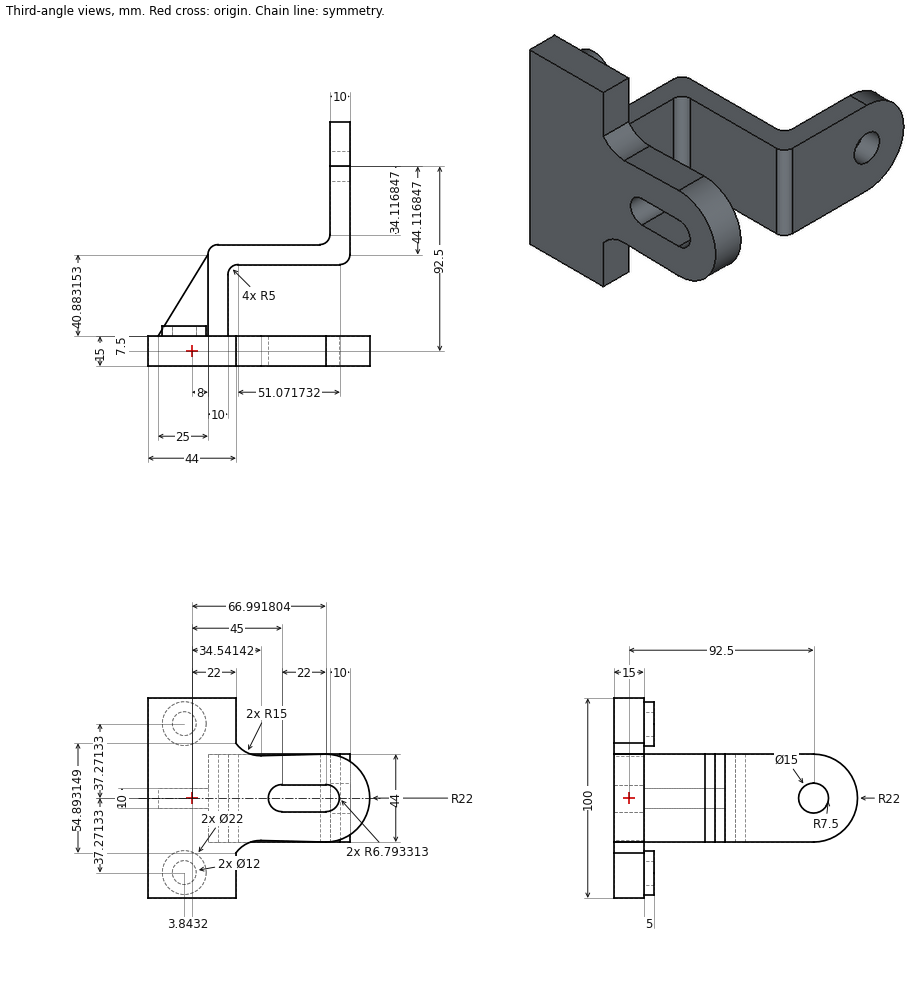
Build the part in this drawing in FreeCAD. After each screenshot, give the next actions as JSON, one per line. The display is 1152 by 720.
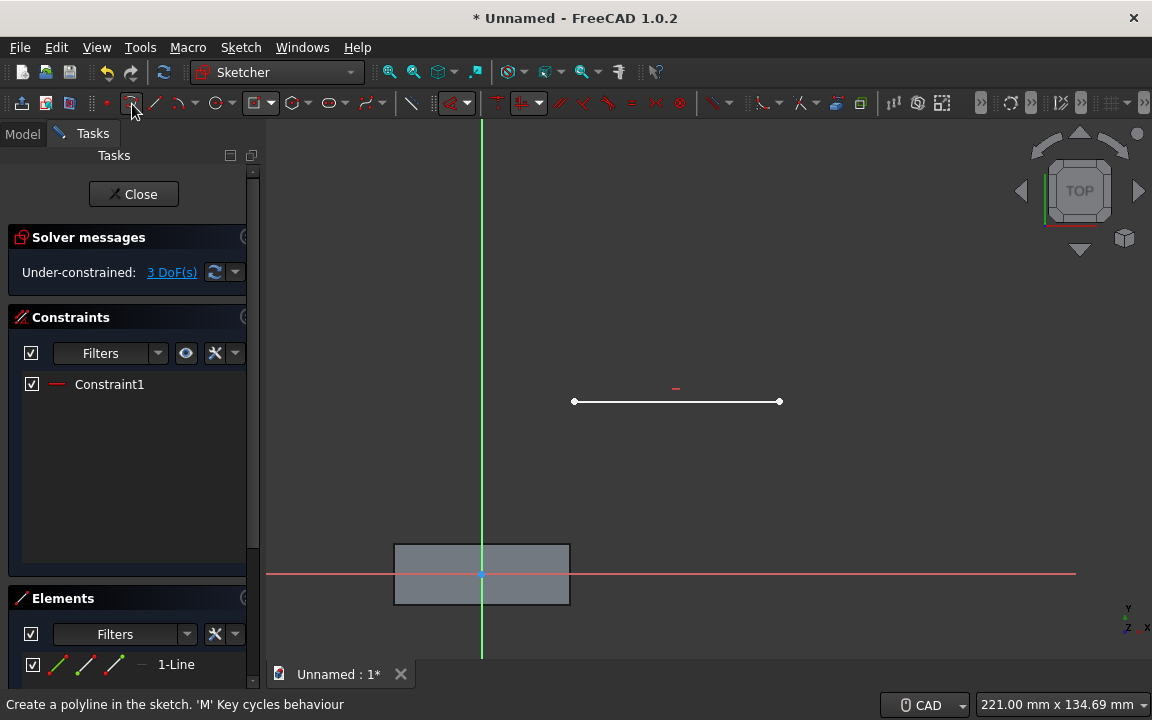
{"action": "left_click", "coordinate": [799, 380]}
{"action": "left_click", "coordinate": [799, 204]}
{"action": "left_click", "coordinate": [759, 204]}
{"action": "left_click", "coordinate": [759, 340]}
{"action": "right_click", "coordinate": [759, 340]}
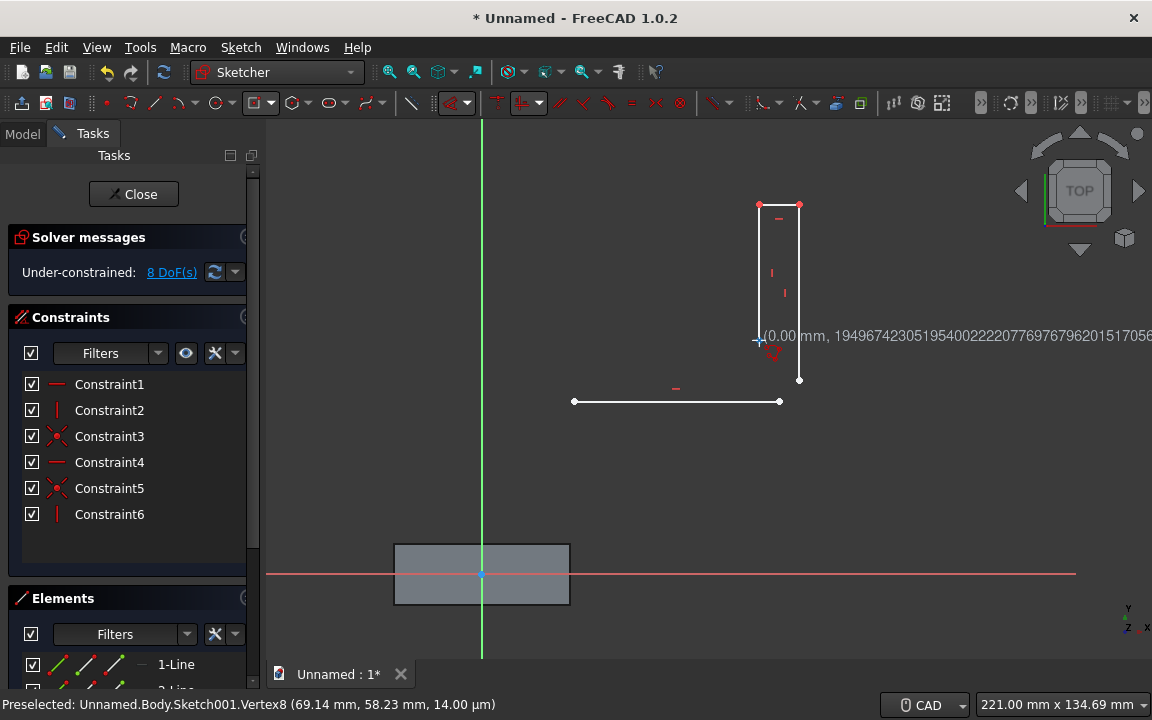
{"action": "left_click", "coordinate": [156, 104]}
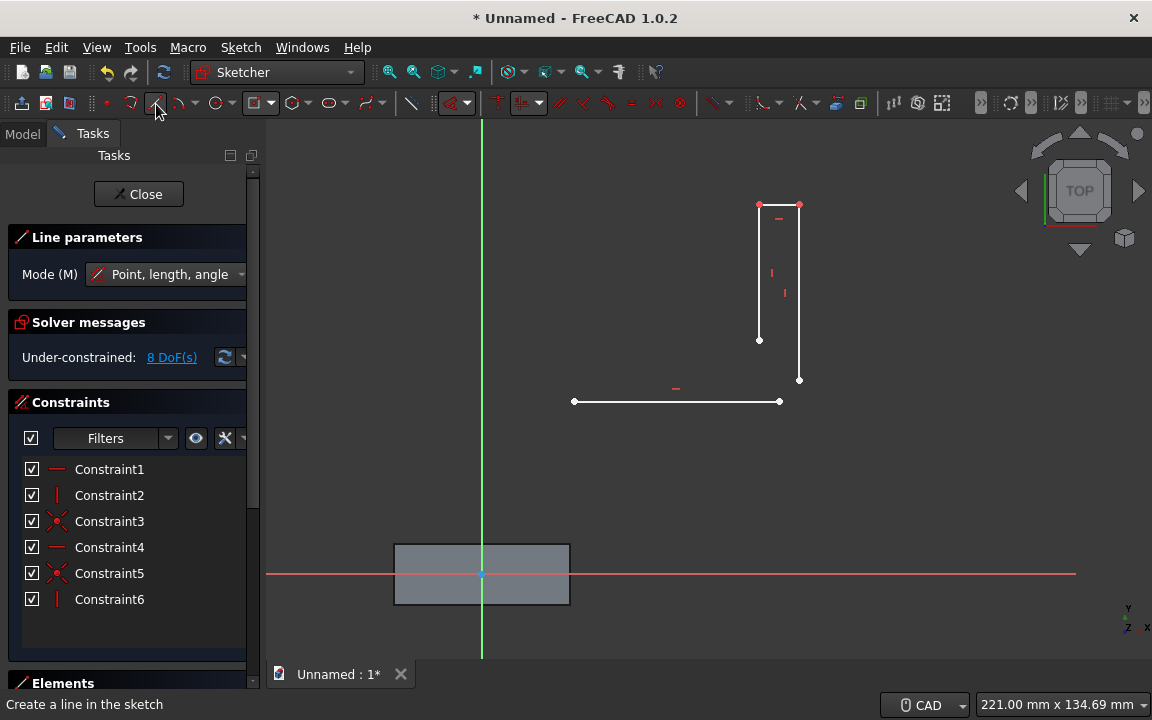
{"action": "left_click", "coordinate": [739, 360]}
{"action": "left_click", "coordinate": [534, 360]}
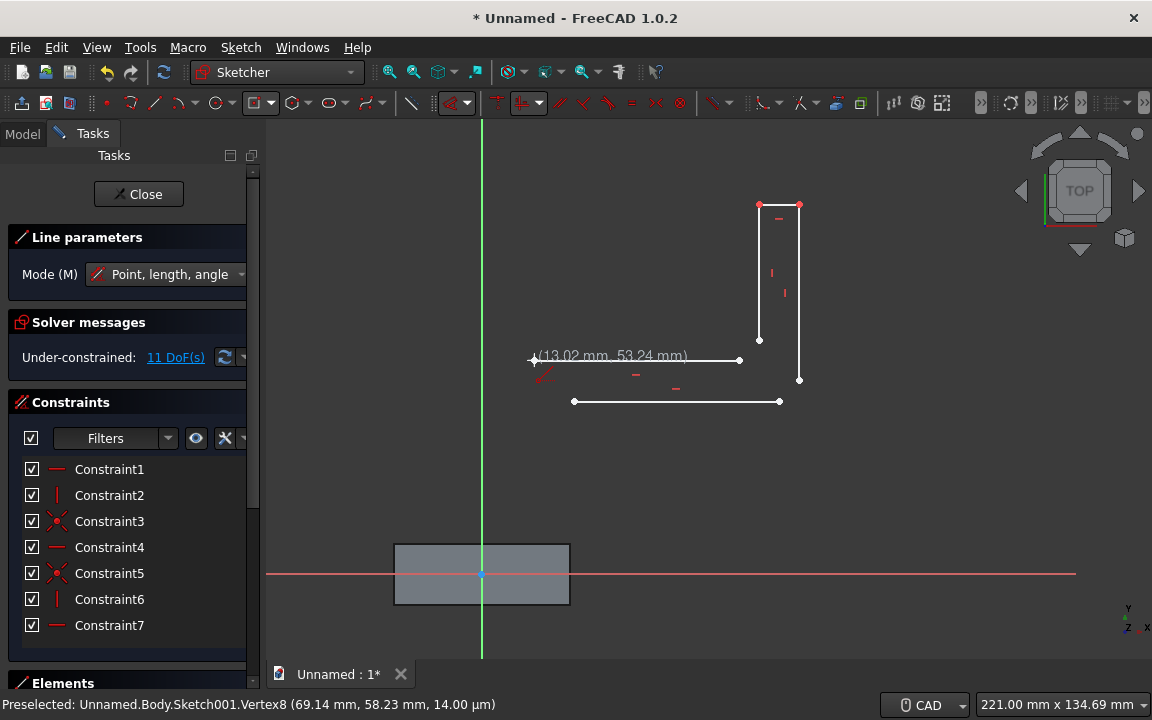
{"action": "left_click", "coordinate": [132, 104]}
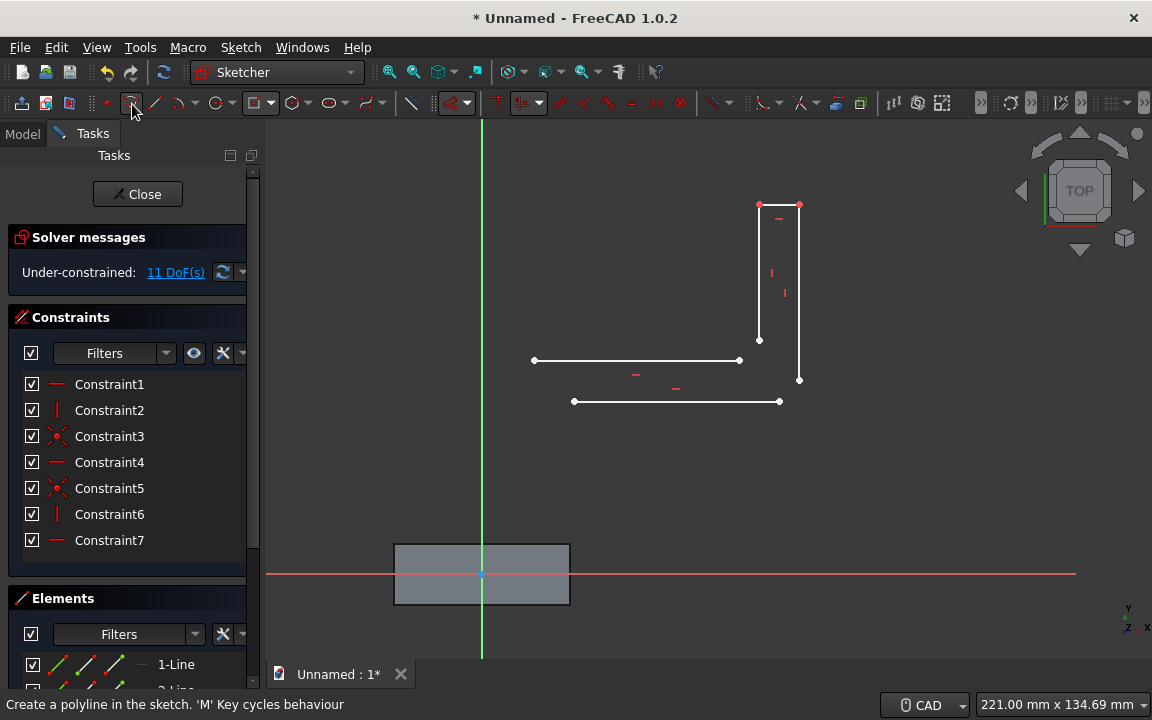
{"action": "left_click", "coordinate": [514, 380]}
{"action": "left_click", "coordinate": [514, 544]}
{"action": "left_click", "coordinate": [554, 544]}
{"action": "left_click", "coordinate": [554, 421]}
{"action": "right_click", "coordinate": [554, 421]}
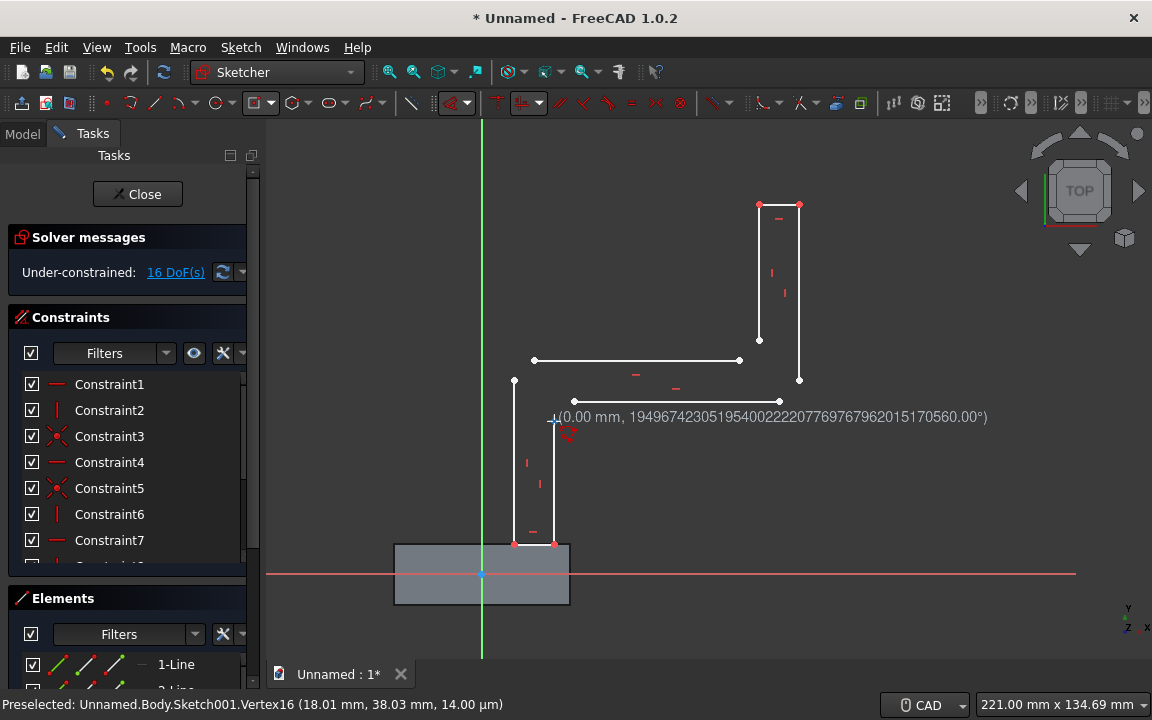
{"action": "left_click", "coordinate": [198, 104]}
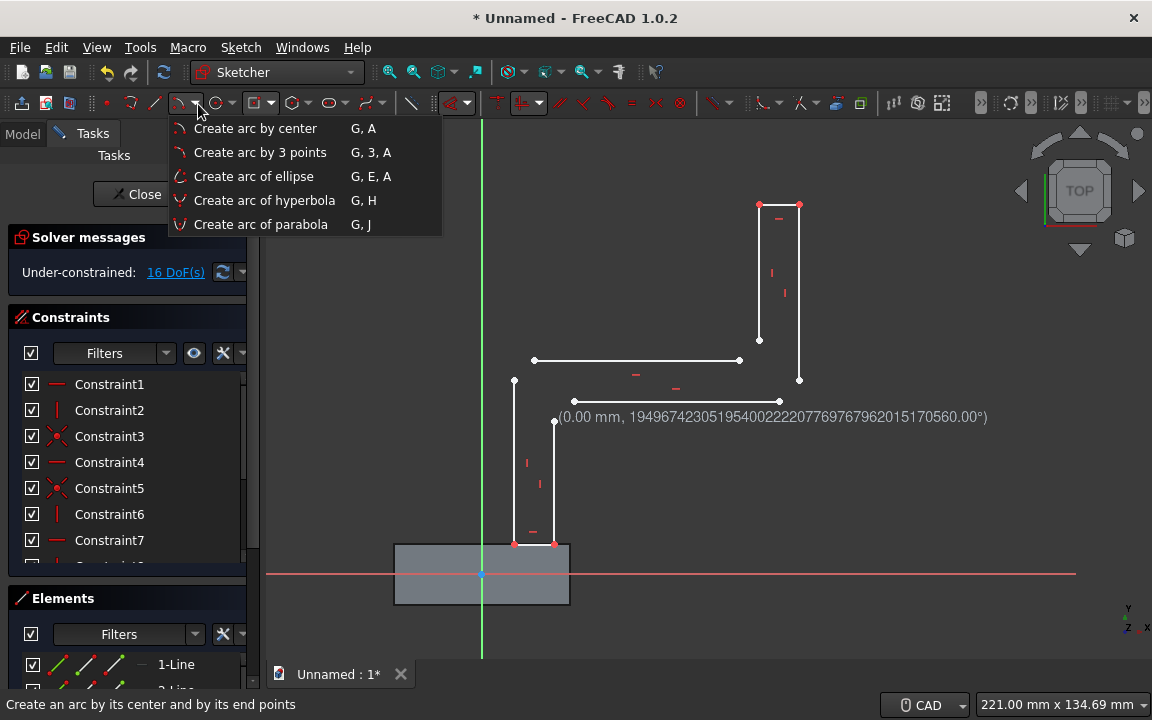
{"action": "left_click", "coordinate": [306, 152]}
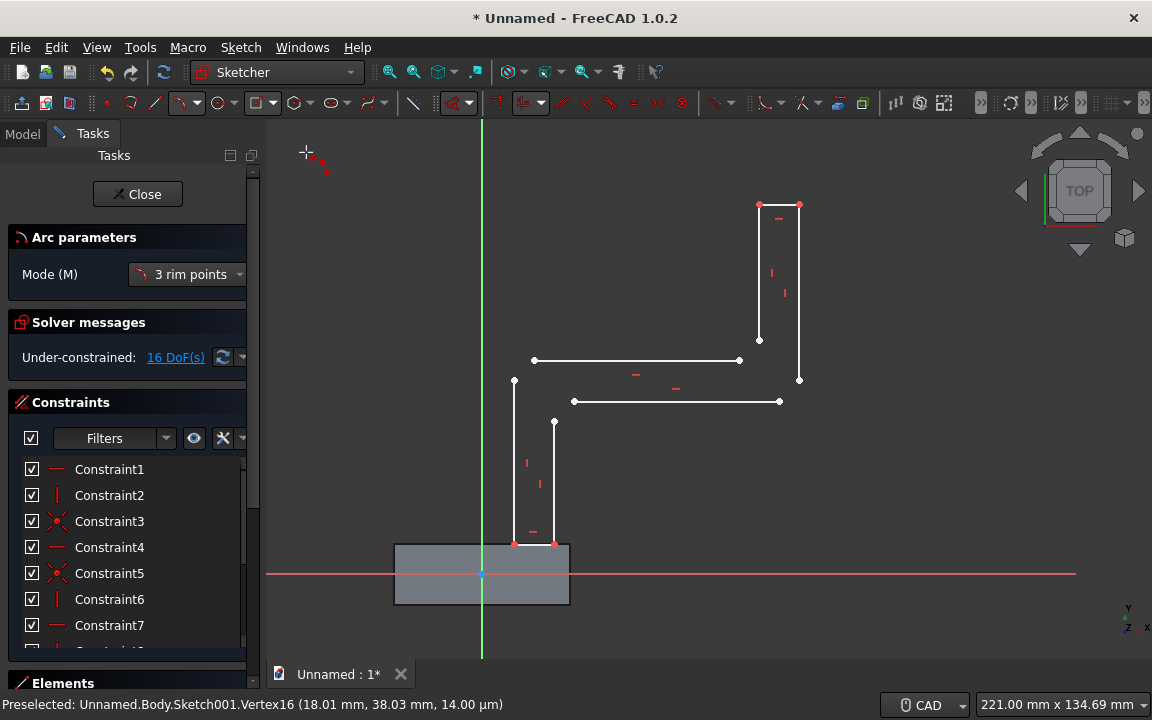
{"action": "left_click", "coordinate": [779, 402]}
{"action": "left_click", "coordinate": [799, 381]}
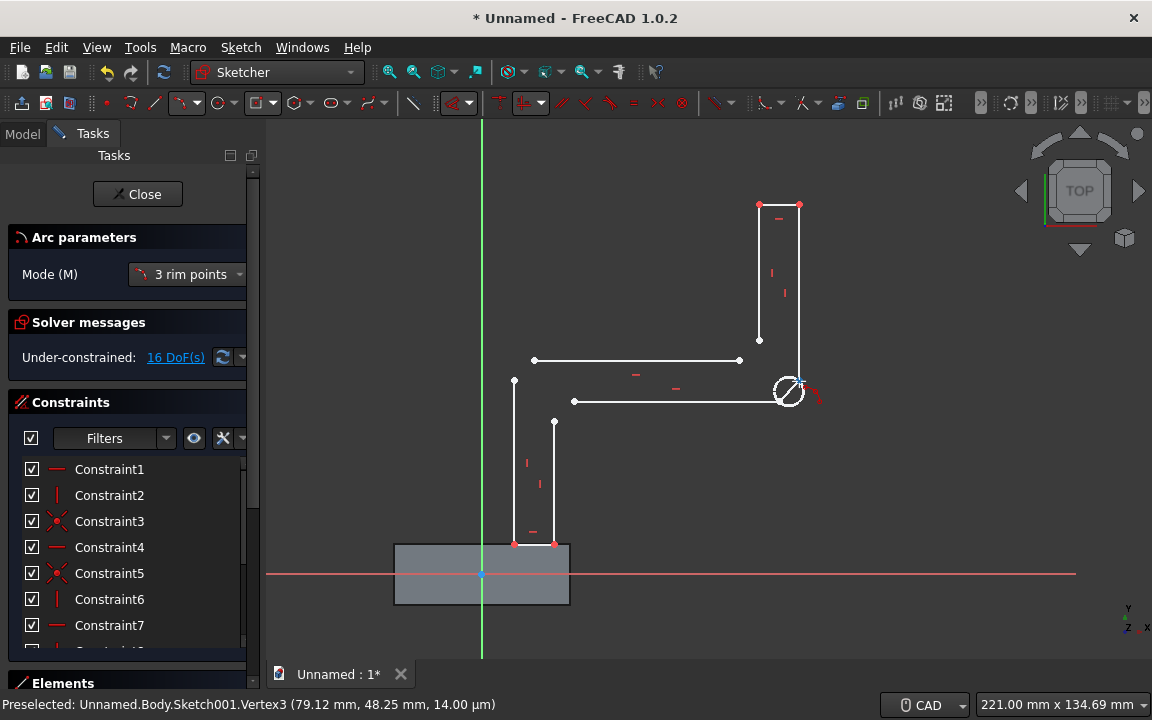
{"action": "scroll", "coordinate": [793, 395], "scroll_direction": "up", "scroll_amount": 5}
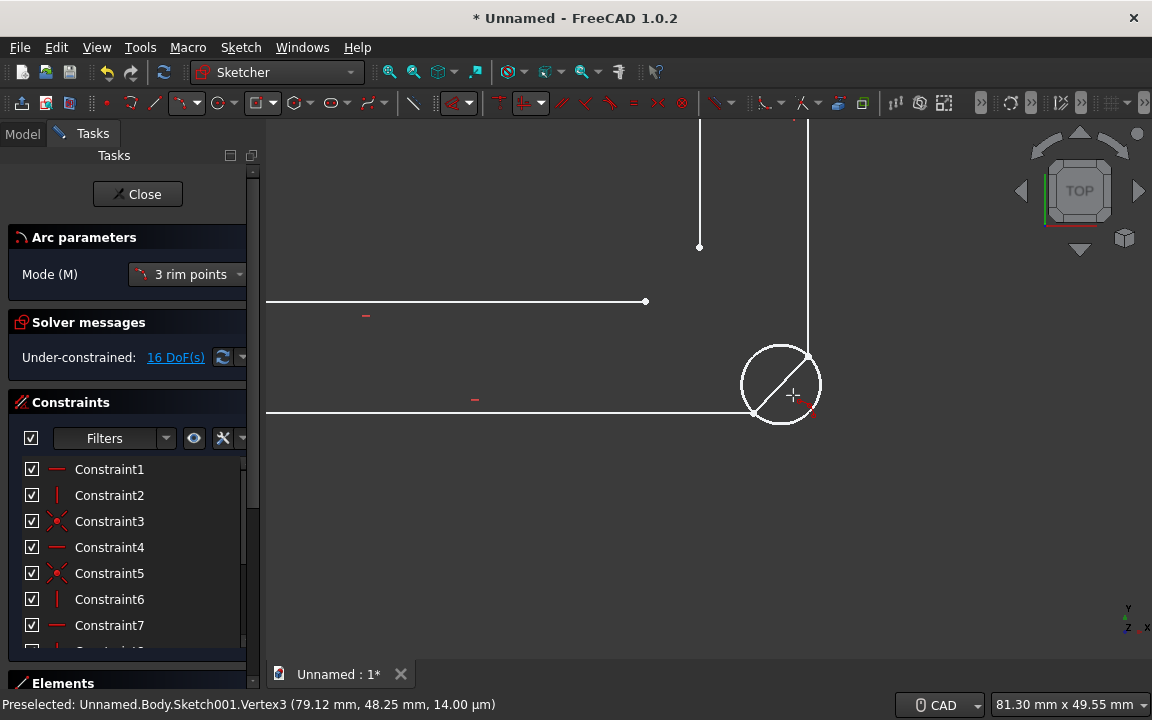
{"action": "left_click", "coordinate": [792, 393]}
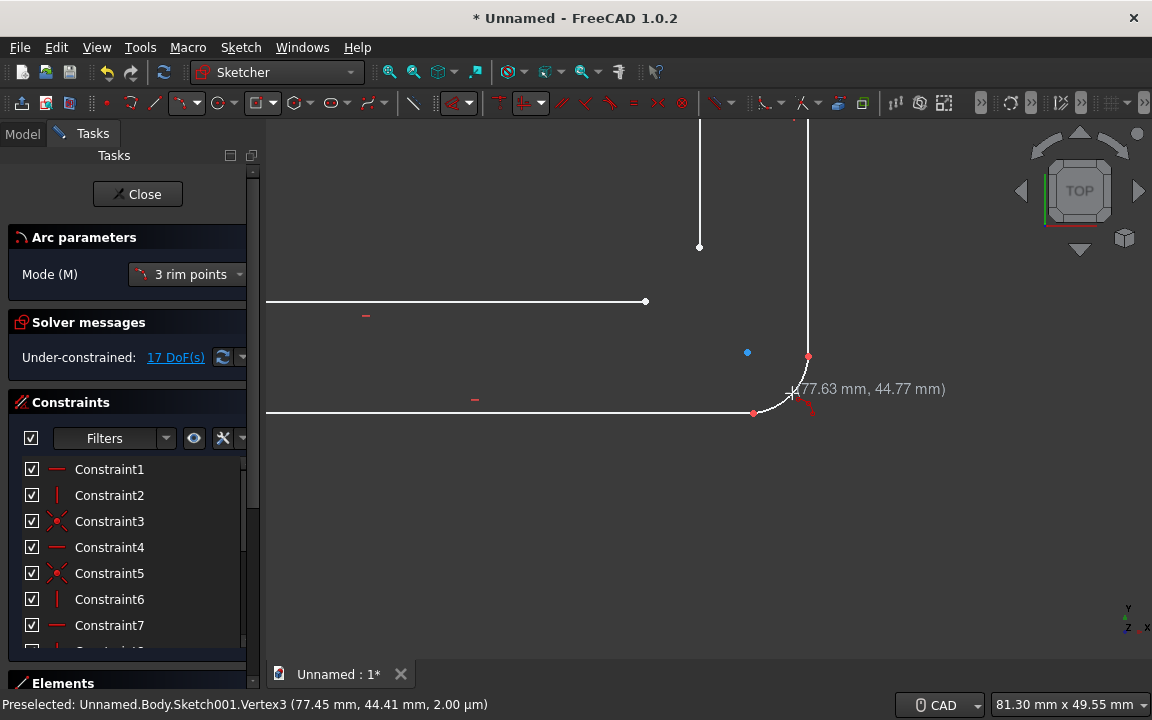
{"action": "left_click", "coordinate": [700, 247]}
{"action": "left_click", "coordinate": [645, 302]}
{"action": "left_click", "coordinate": [683, 284]}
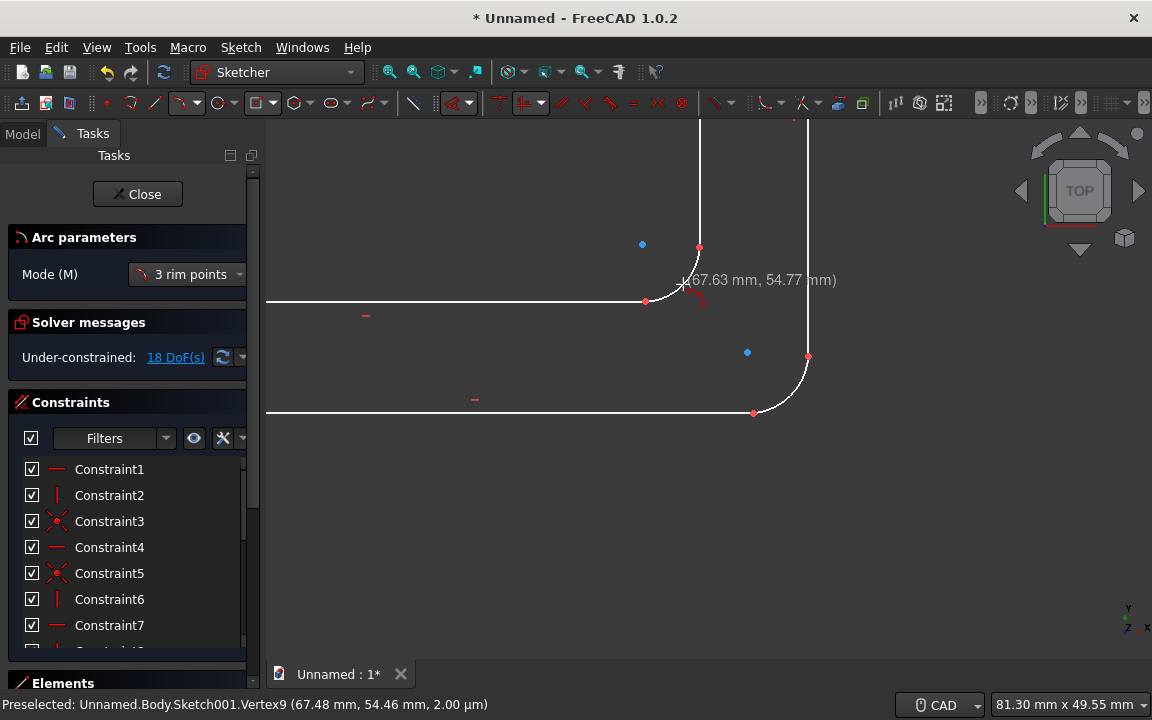
{"action": "scroll", "coordinate": [794, 395], "scroll_direction": "down", "scroll_amount": 5}